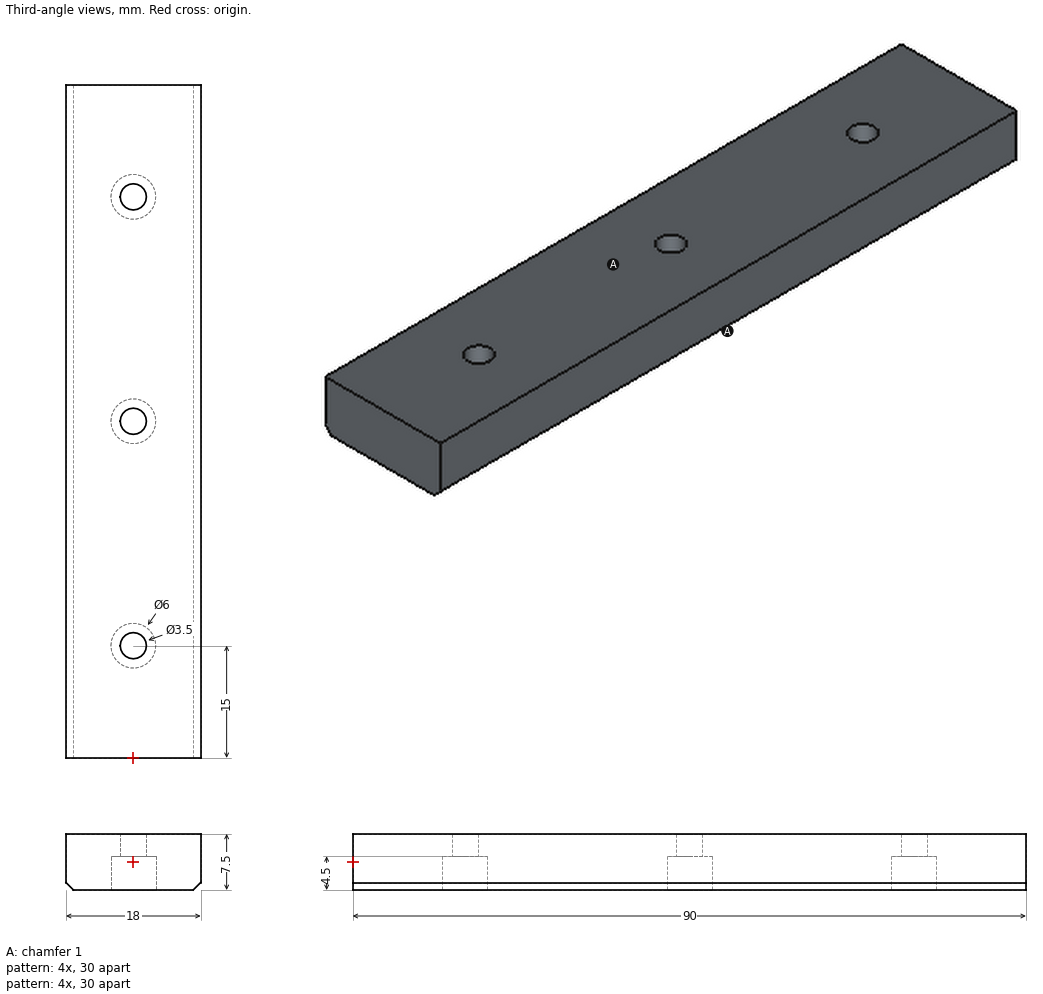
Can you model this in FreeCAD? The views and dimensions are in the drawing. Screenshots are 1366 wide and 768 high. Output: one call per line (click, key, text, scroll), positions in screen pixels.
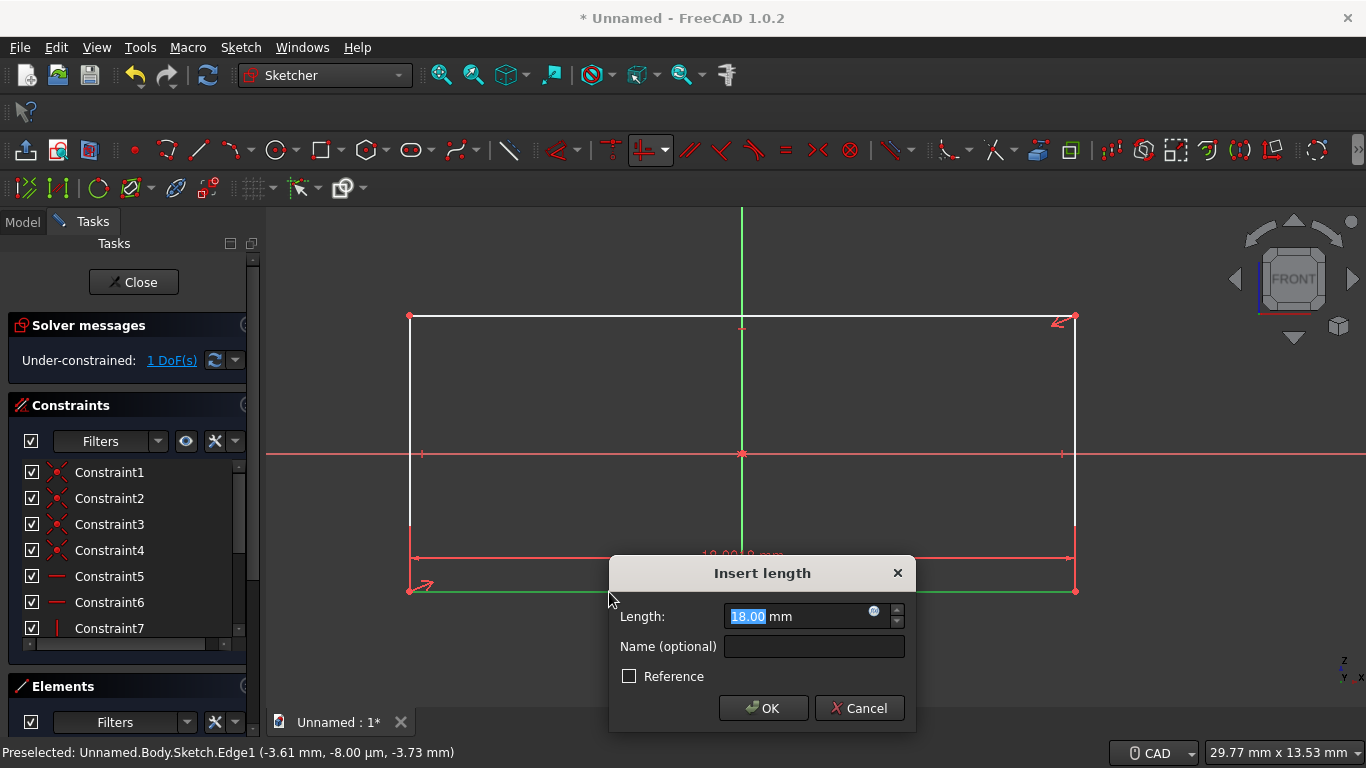
text(18)
key(Return)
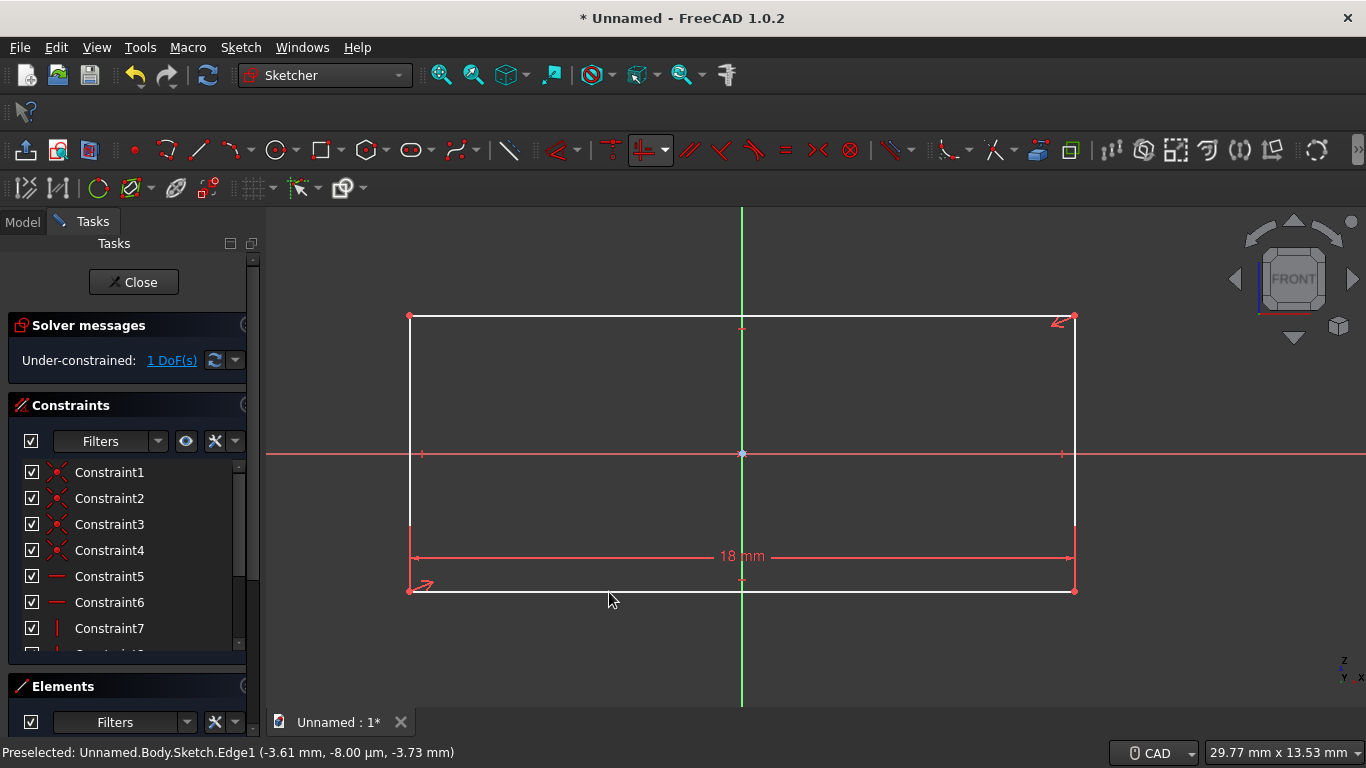
click(1075, 509)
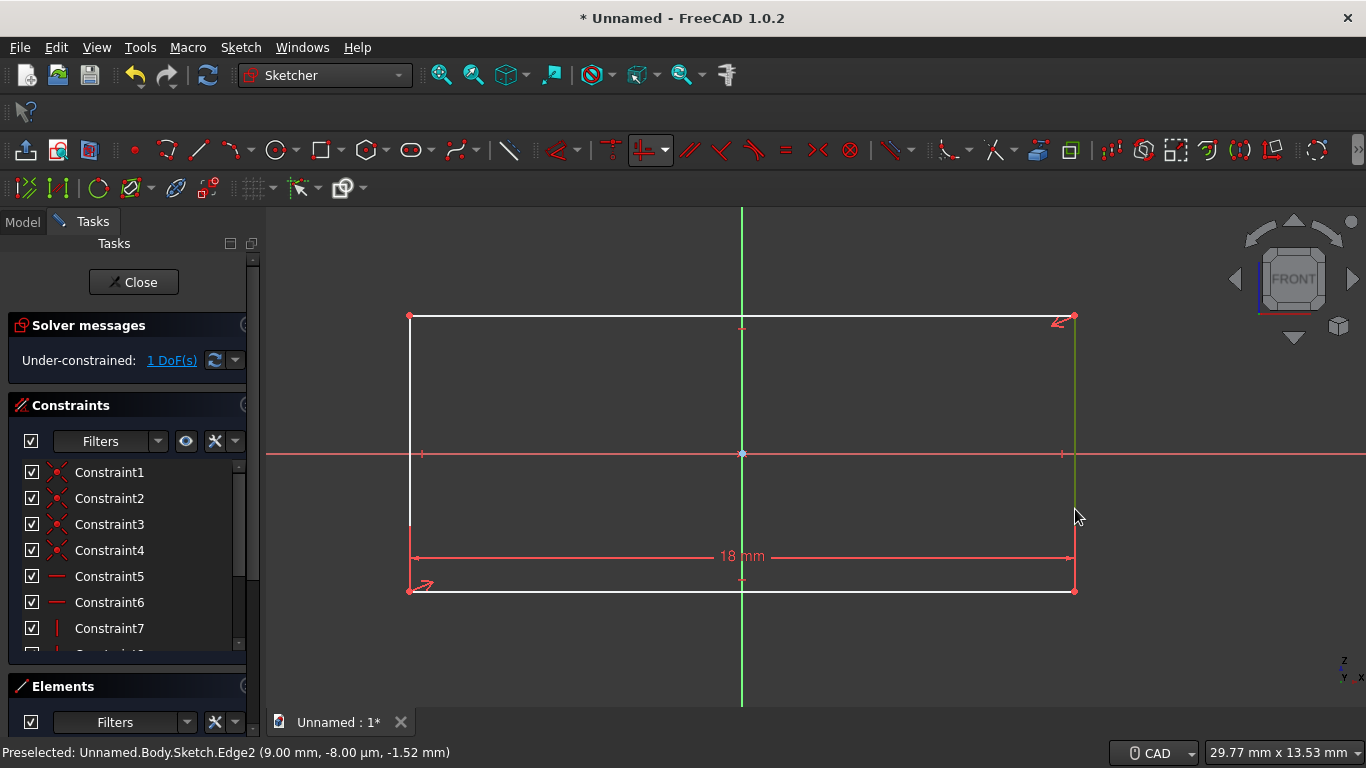
key(i)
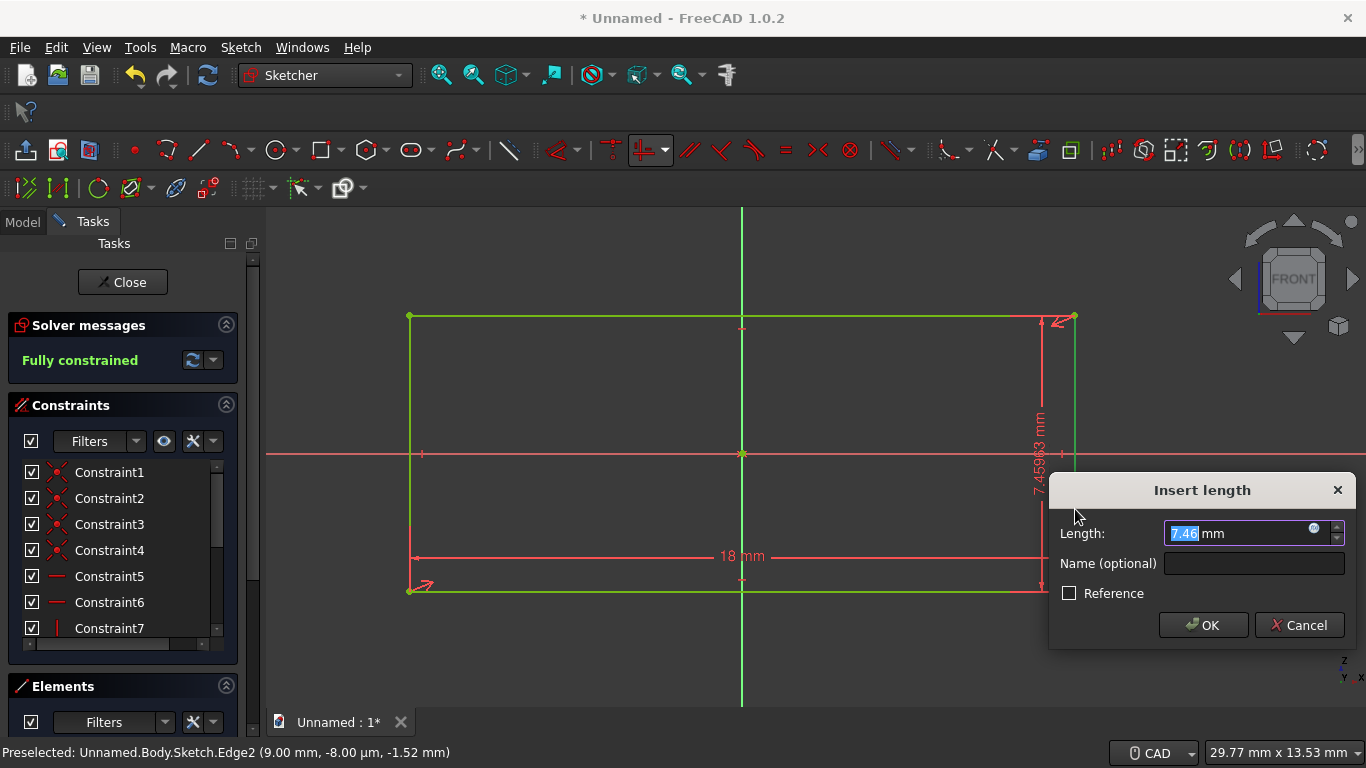
text(7.5)
key(Return)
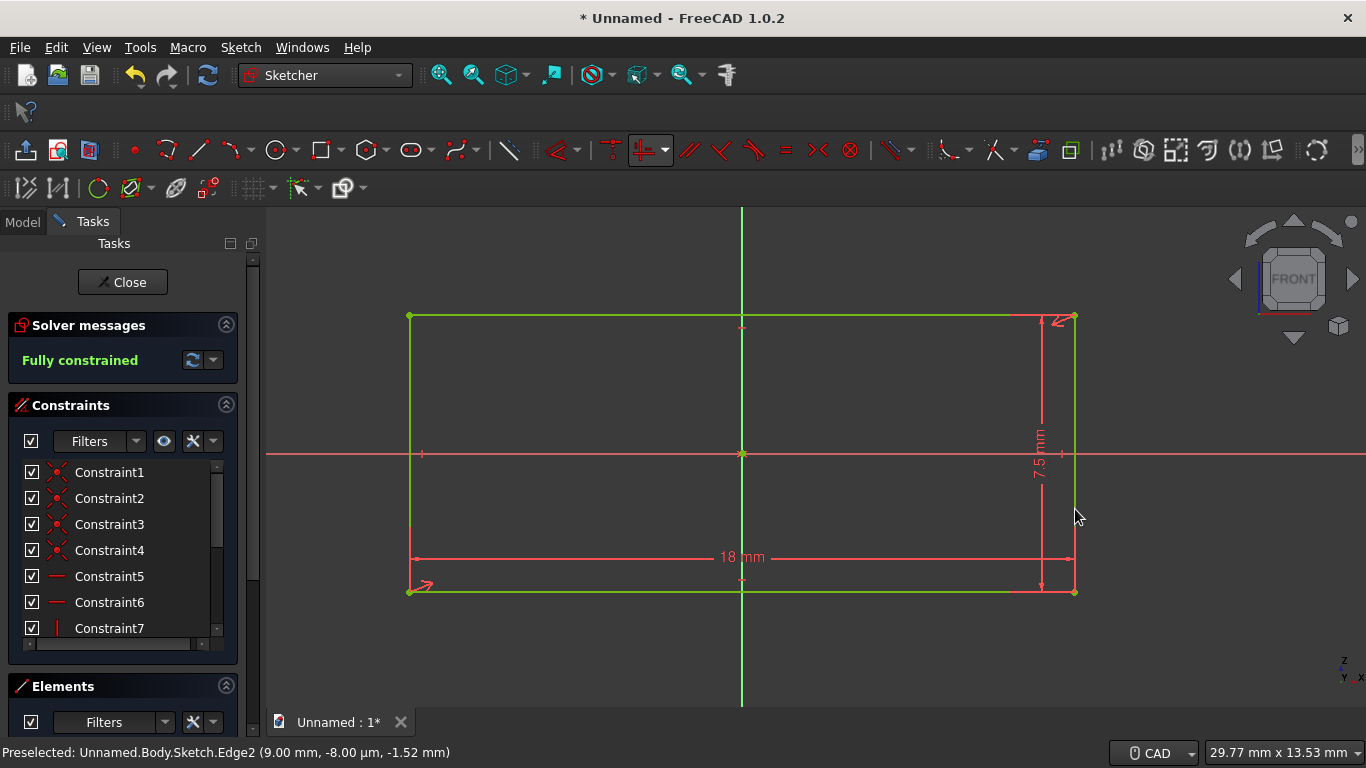
click(123, 282)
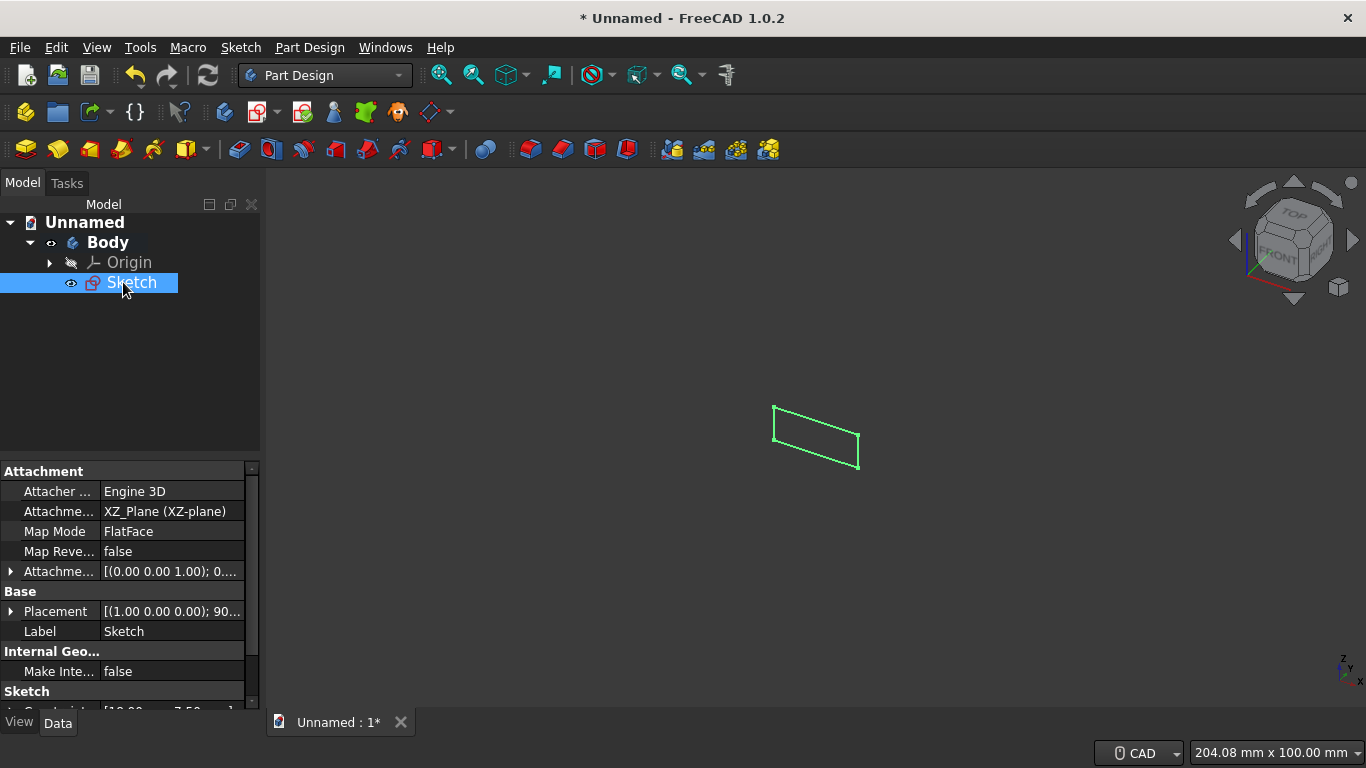
click(26, 150)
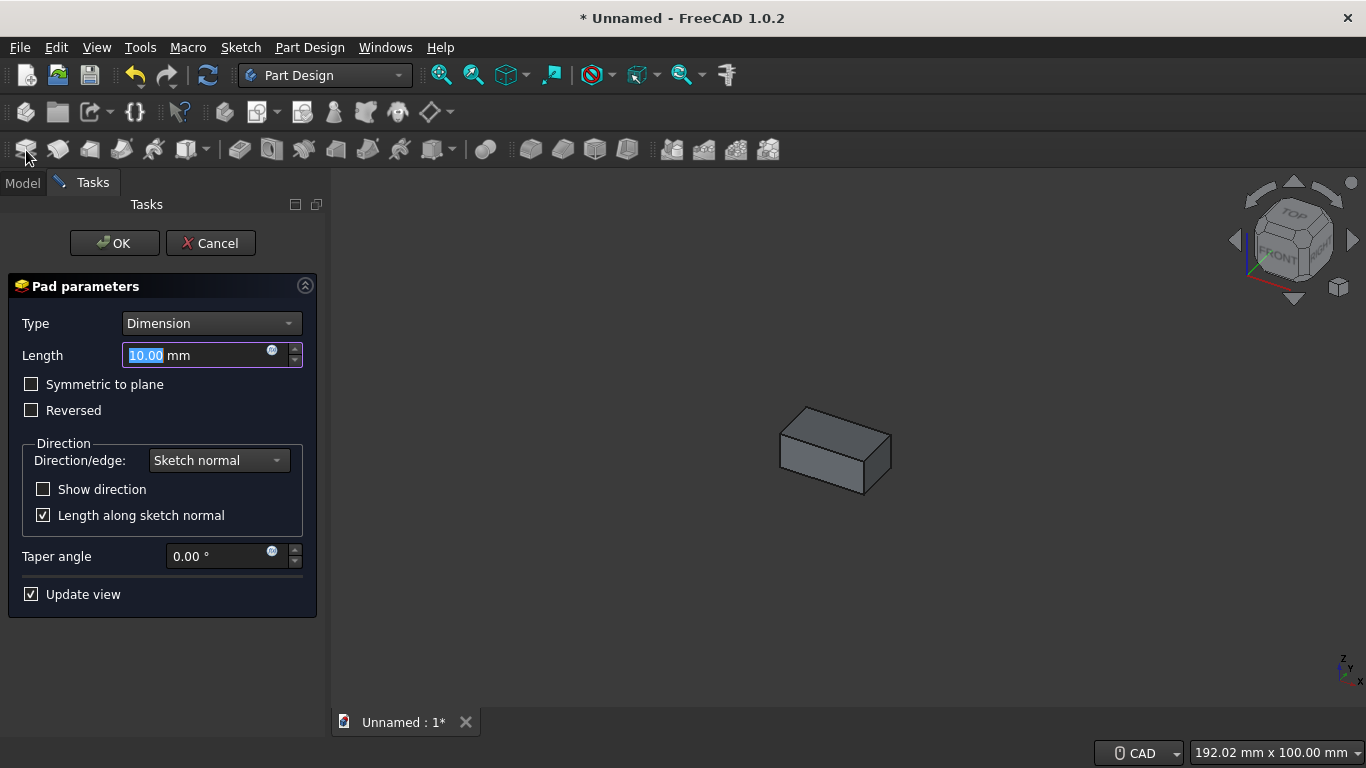
text(90)
key(Tab)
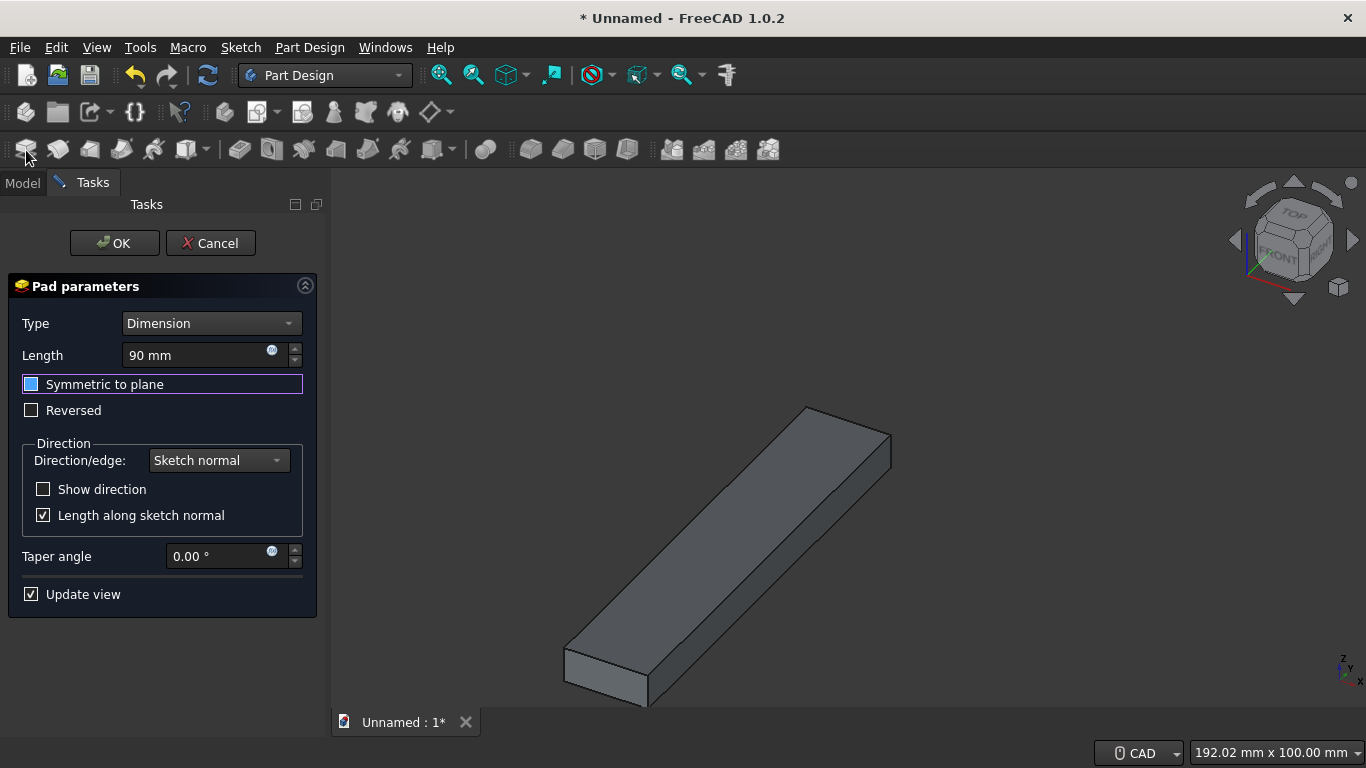
click(30, 410)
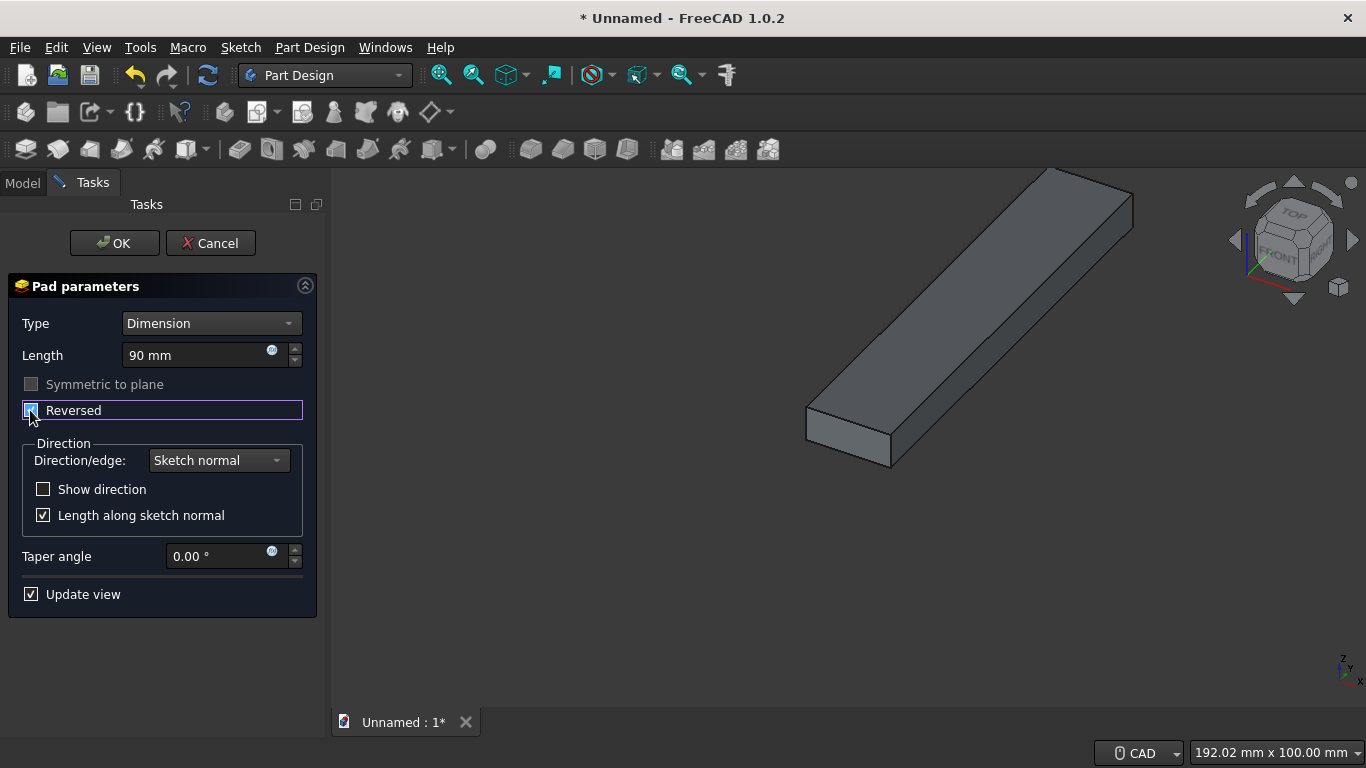
click(115, 243)